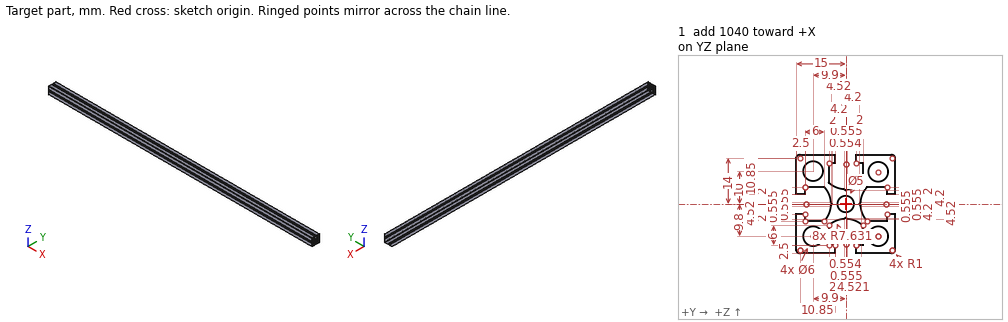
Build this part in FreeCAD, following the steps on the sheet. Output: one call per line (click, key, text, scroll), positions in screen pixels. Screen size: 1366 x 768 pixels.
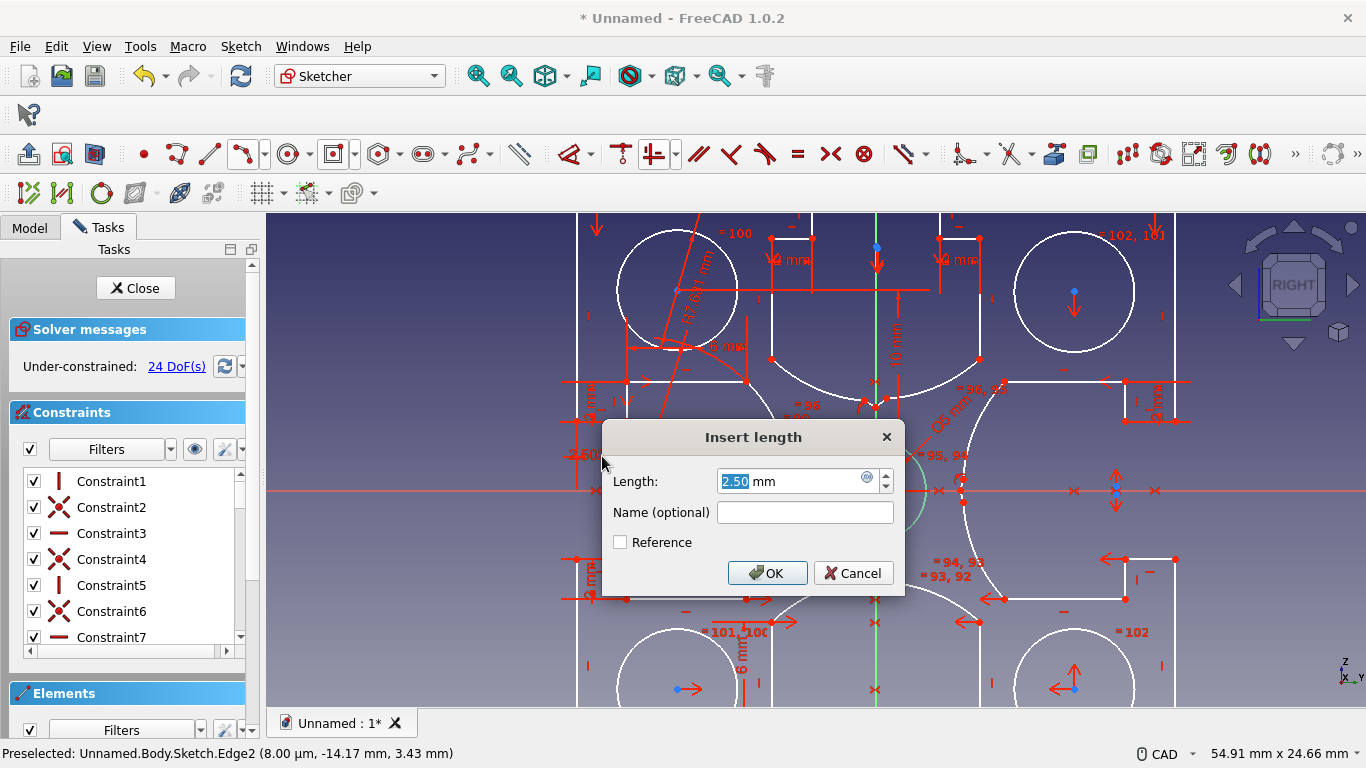
text(2.5)
key(Return)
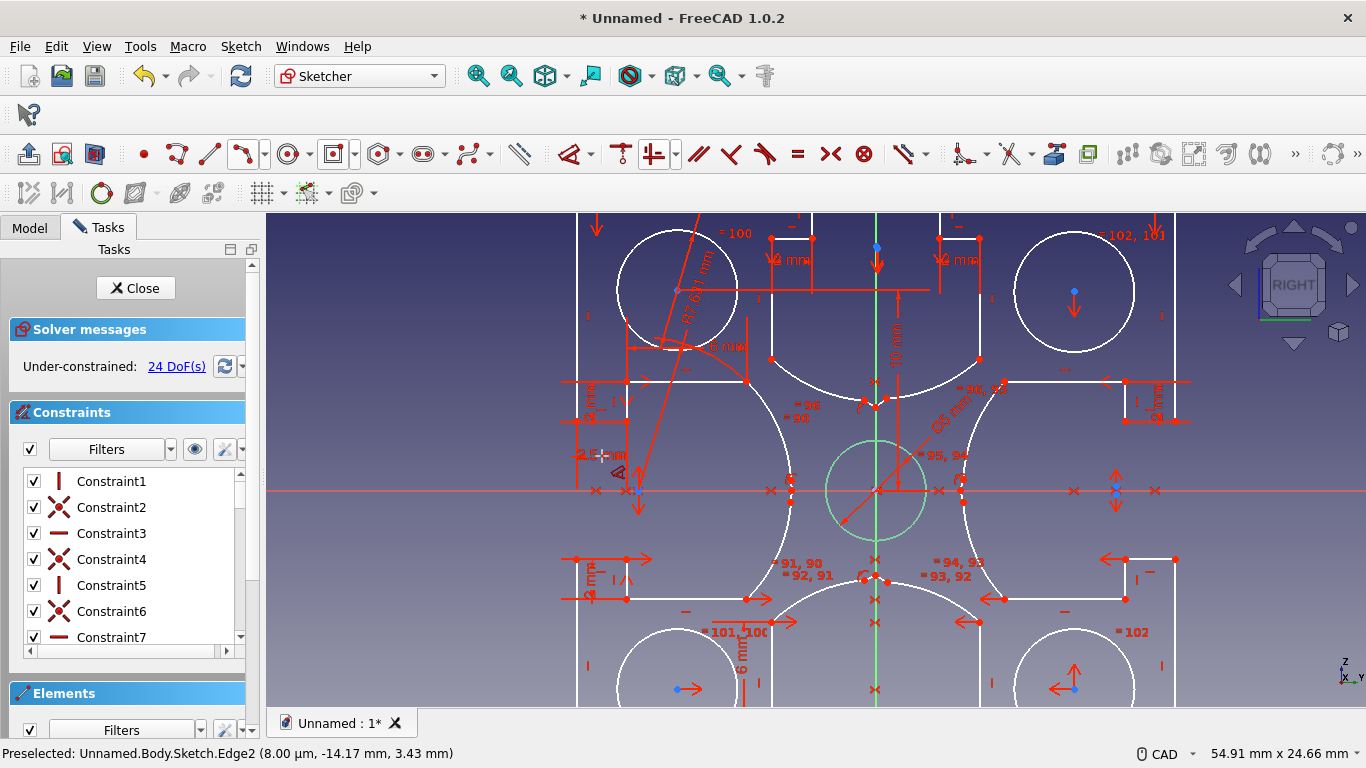
scroll(591, 423, down, 3)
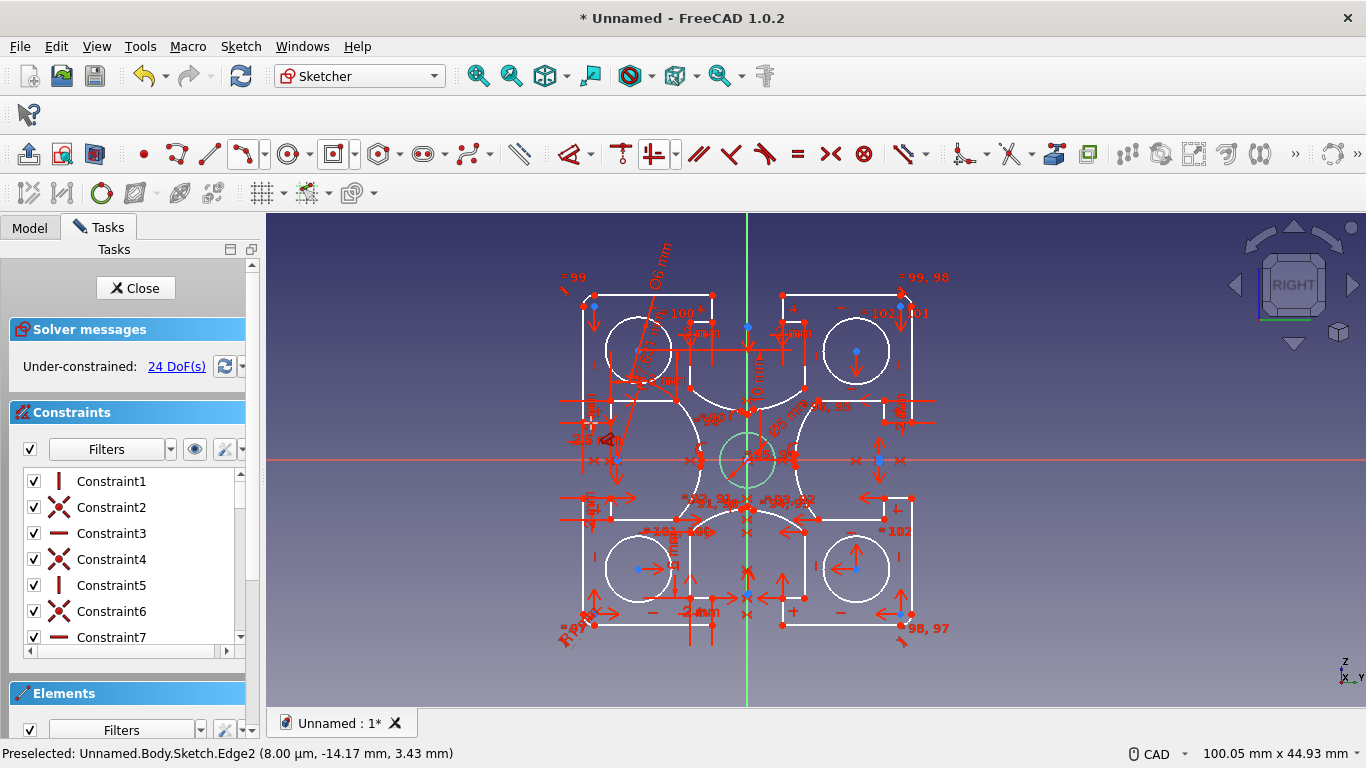
scroll(712, 617, up, 3)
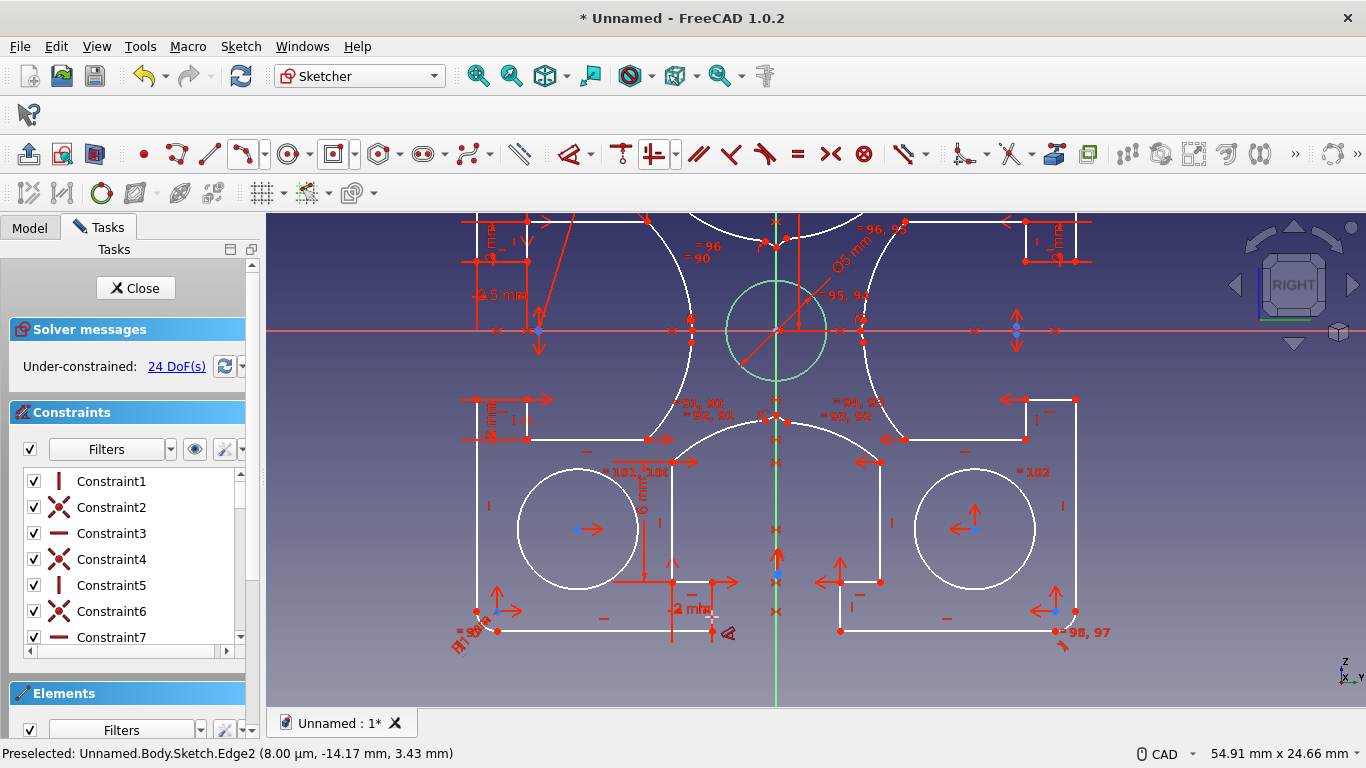
click(712, 617)
click(794, 607)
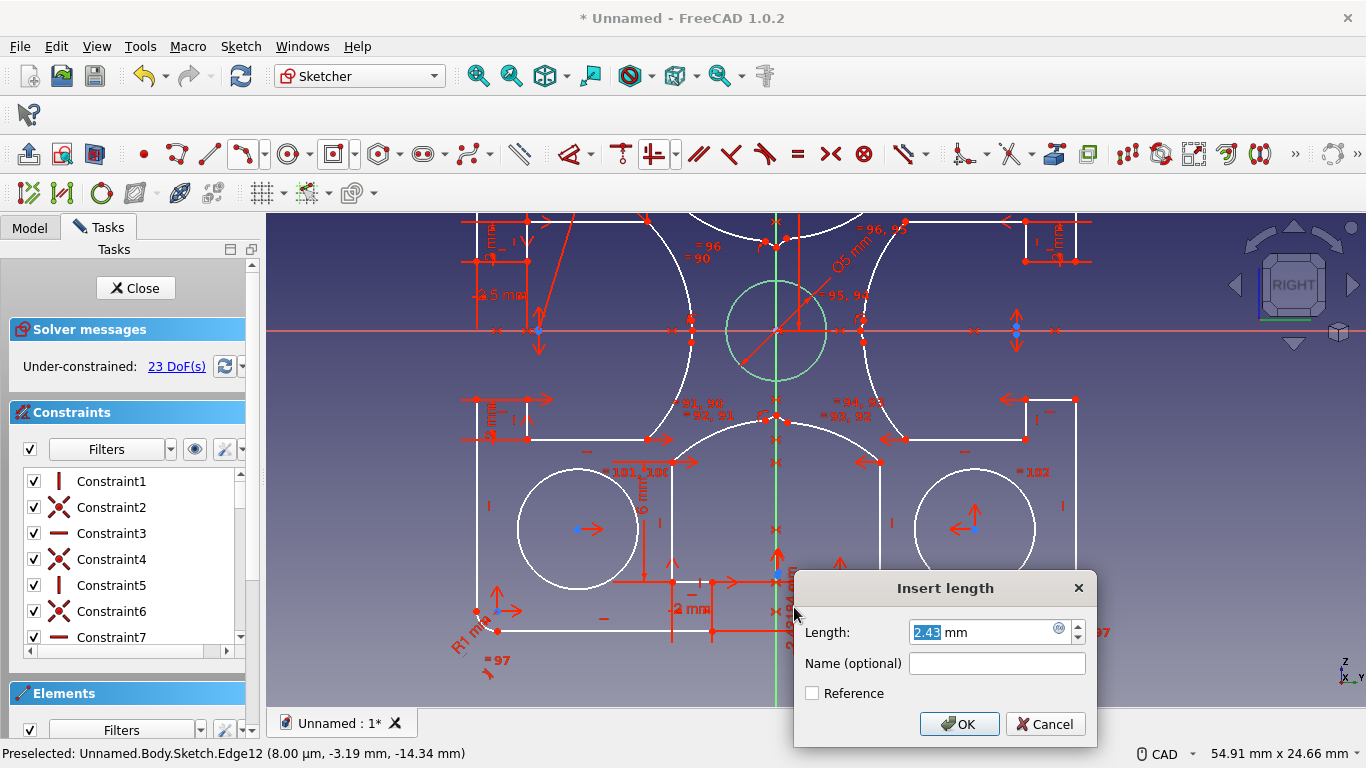
text(2.5)
key(Return)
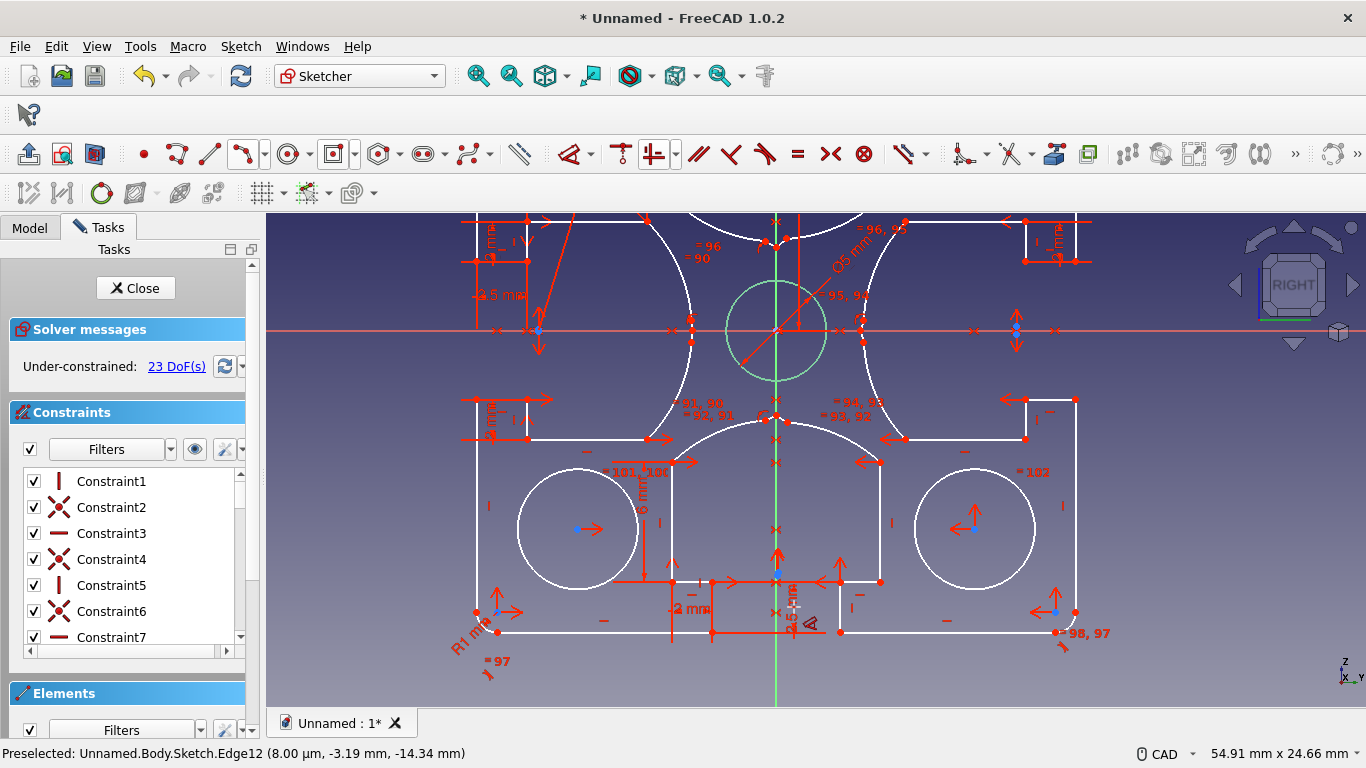
scroll(712, 617, down, 3)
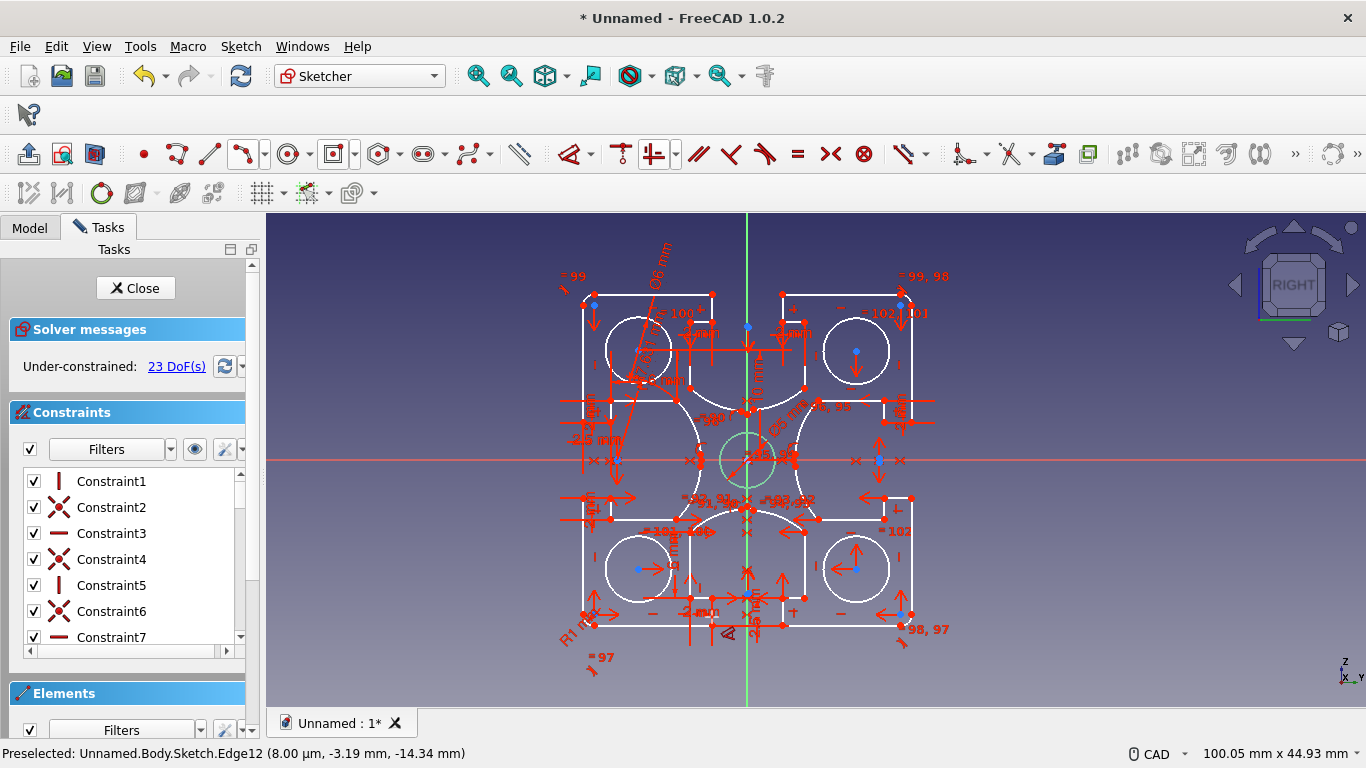
click(583, 306)
click(665, 494)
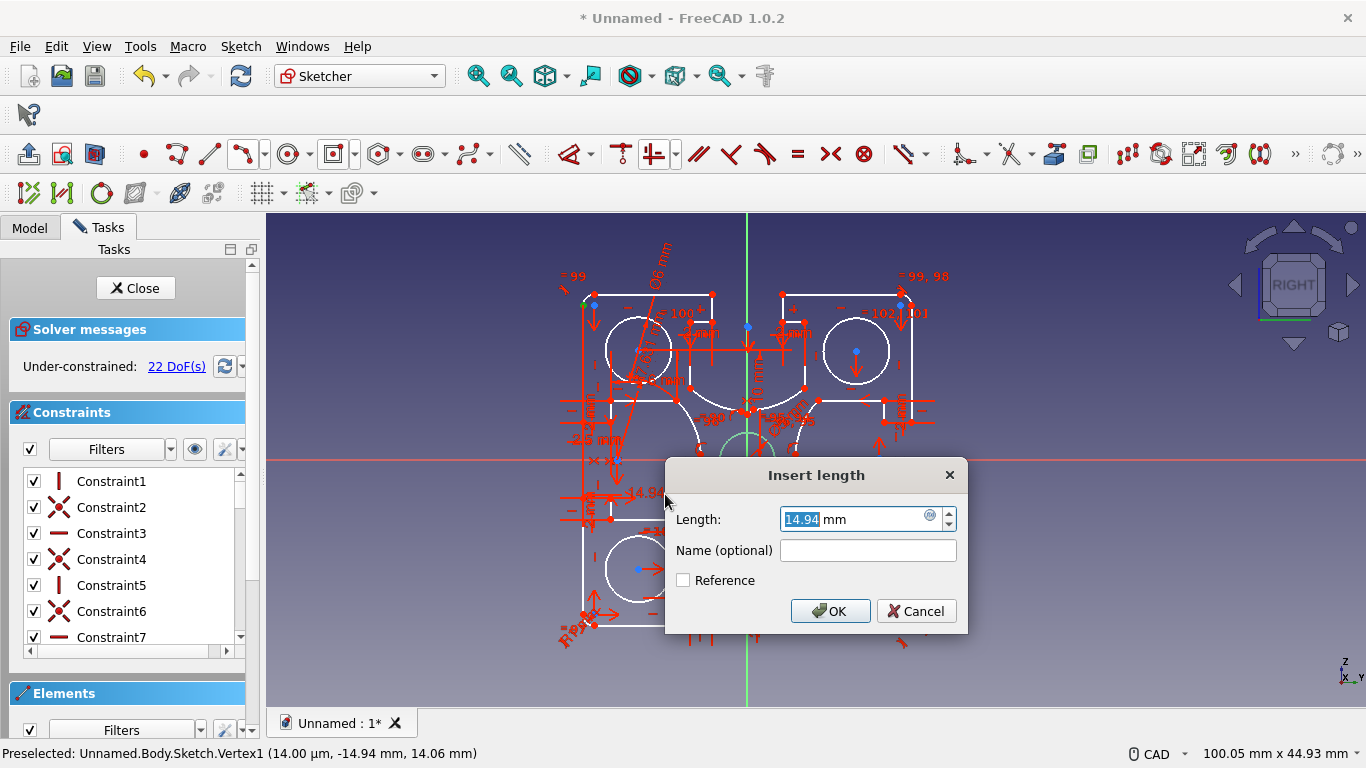
text(15)
key(Return)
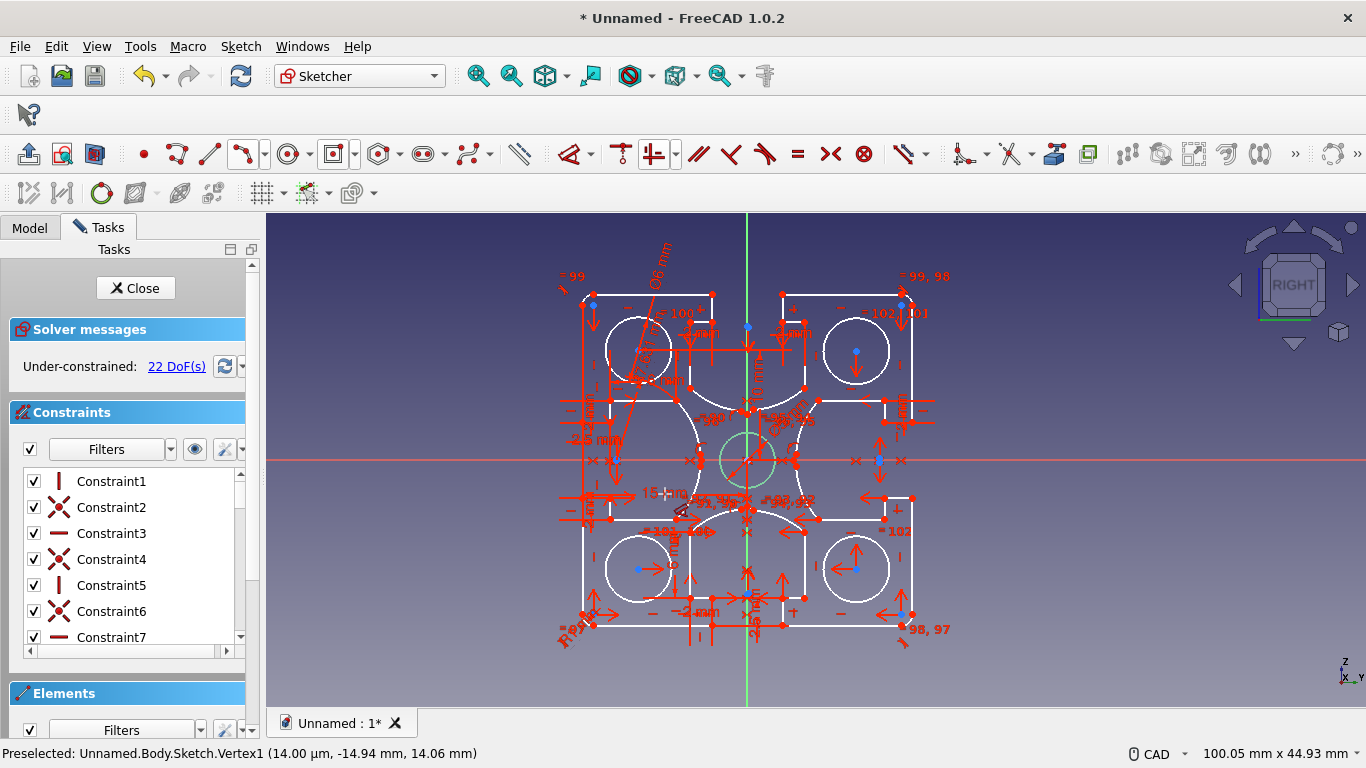
click(583, 306)
click(549, 383)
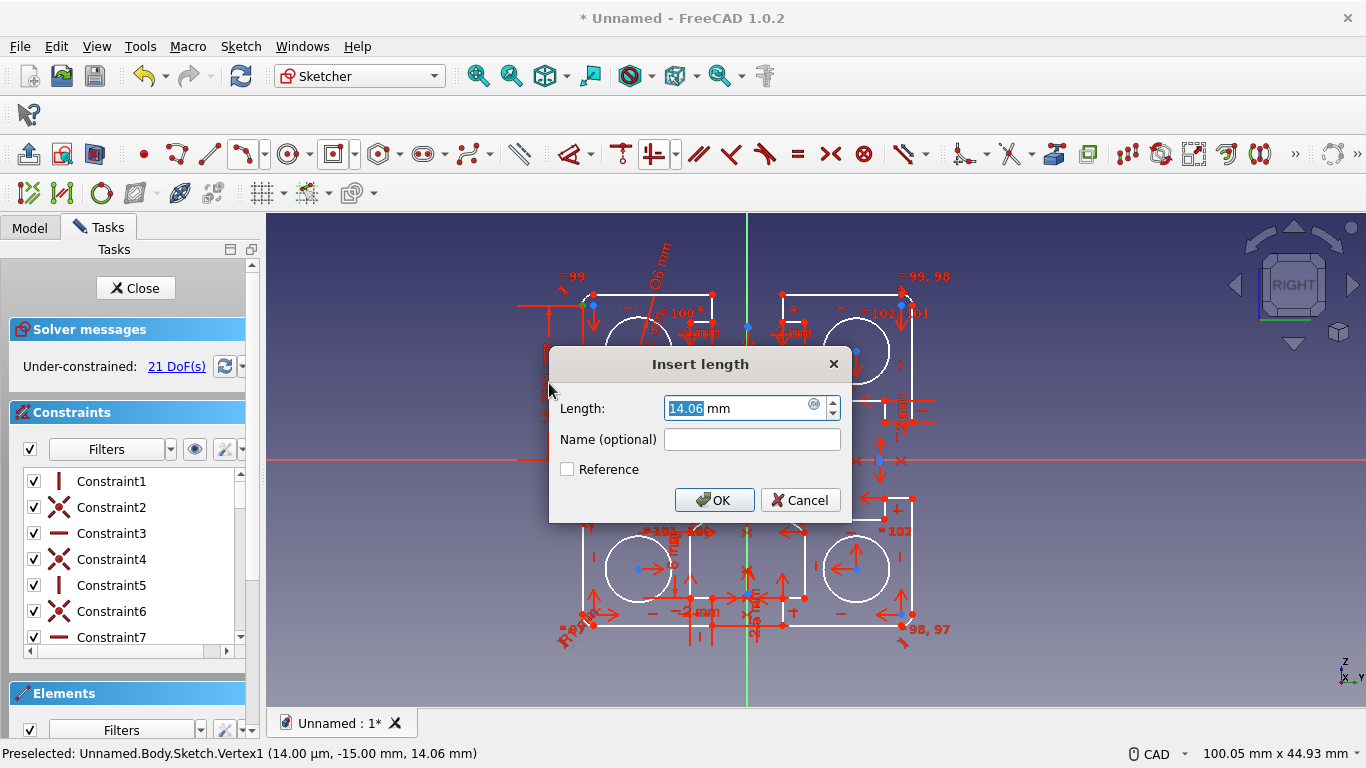
text(14)
key(Return)